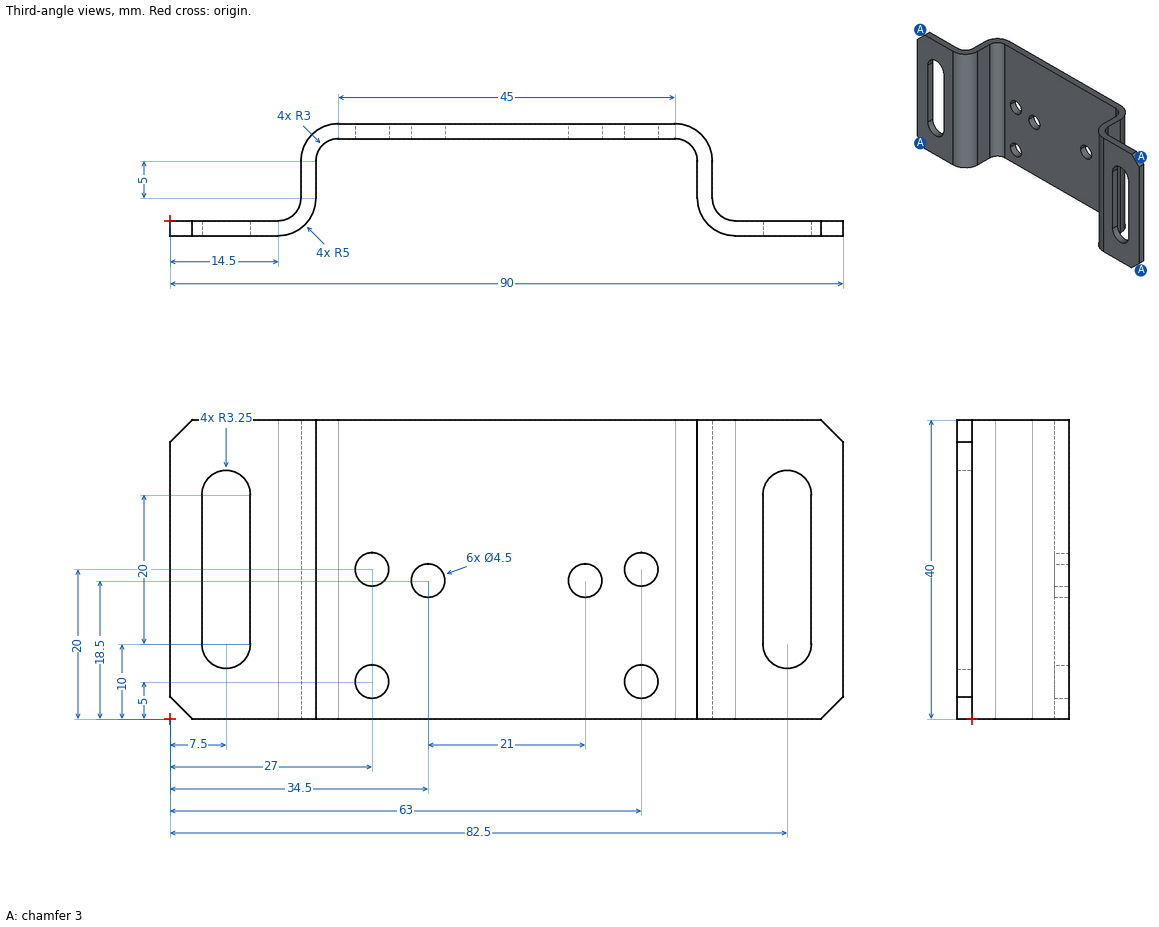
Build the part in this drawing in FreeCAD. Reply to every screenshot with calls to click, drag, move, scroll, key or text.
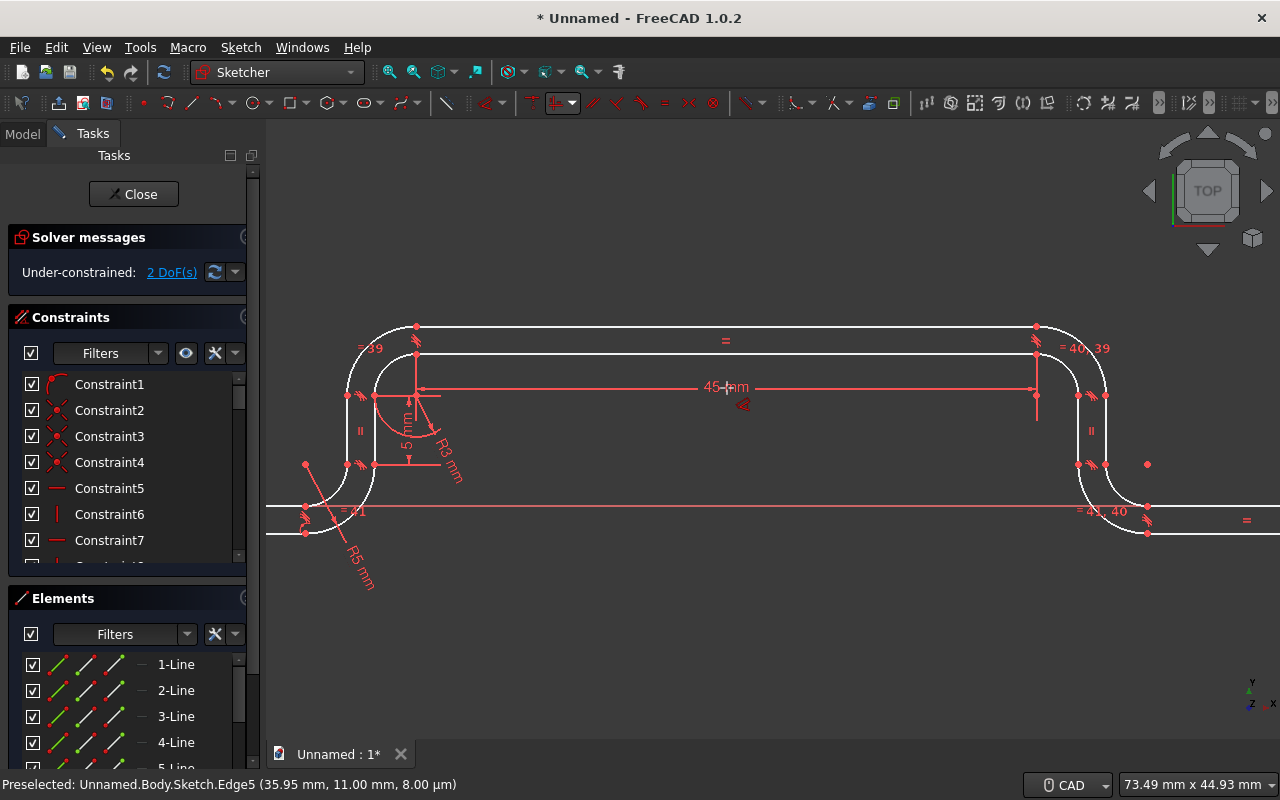
scroll(686, 428, down, 4)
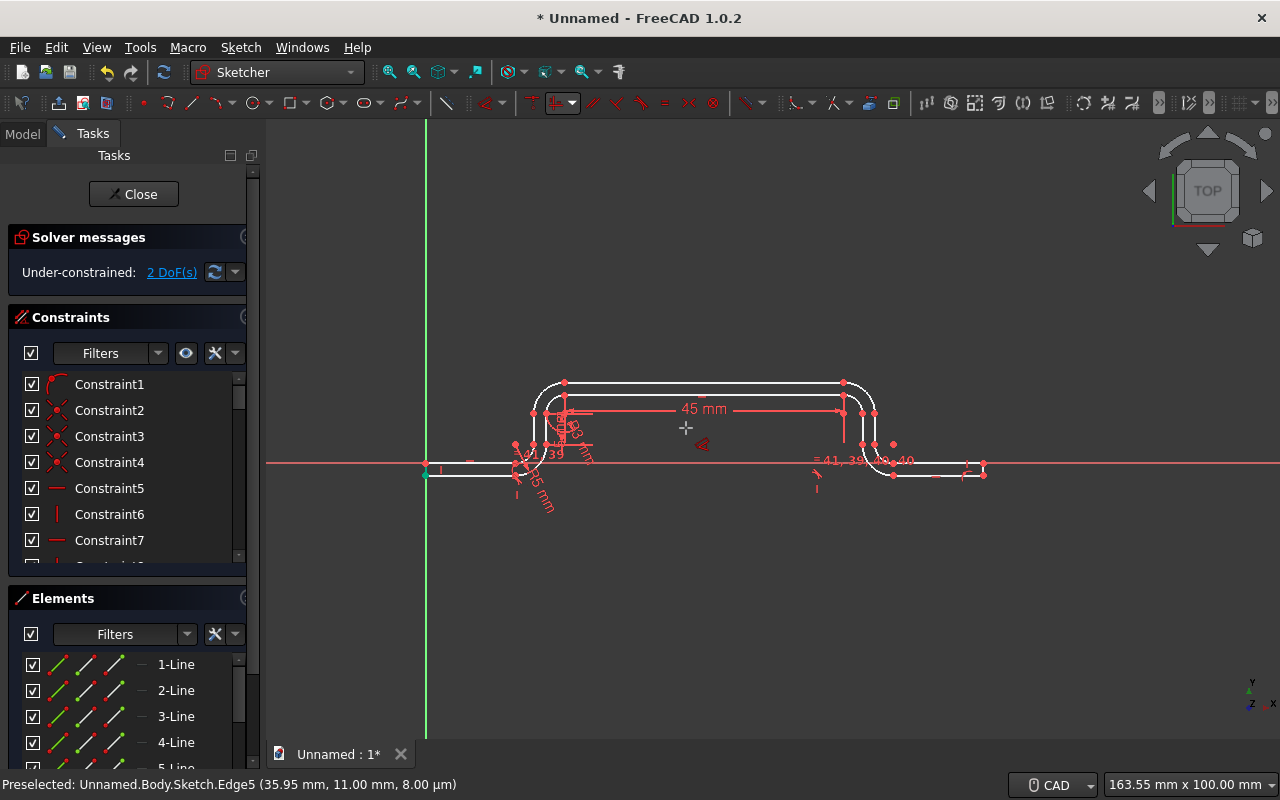
click(983, 476)
click(704, 510)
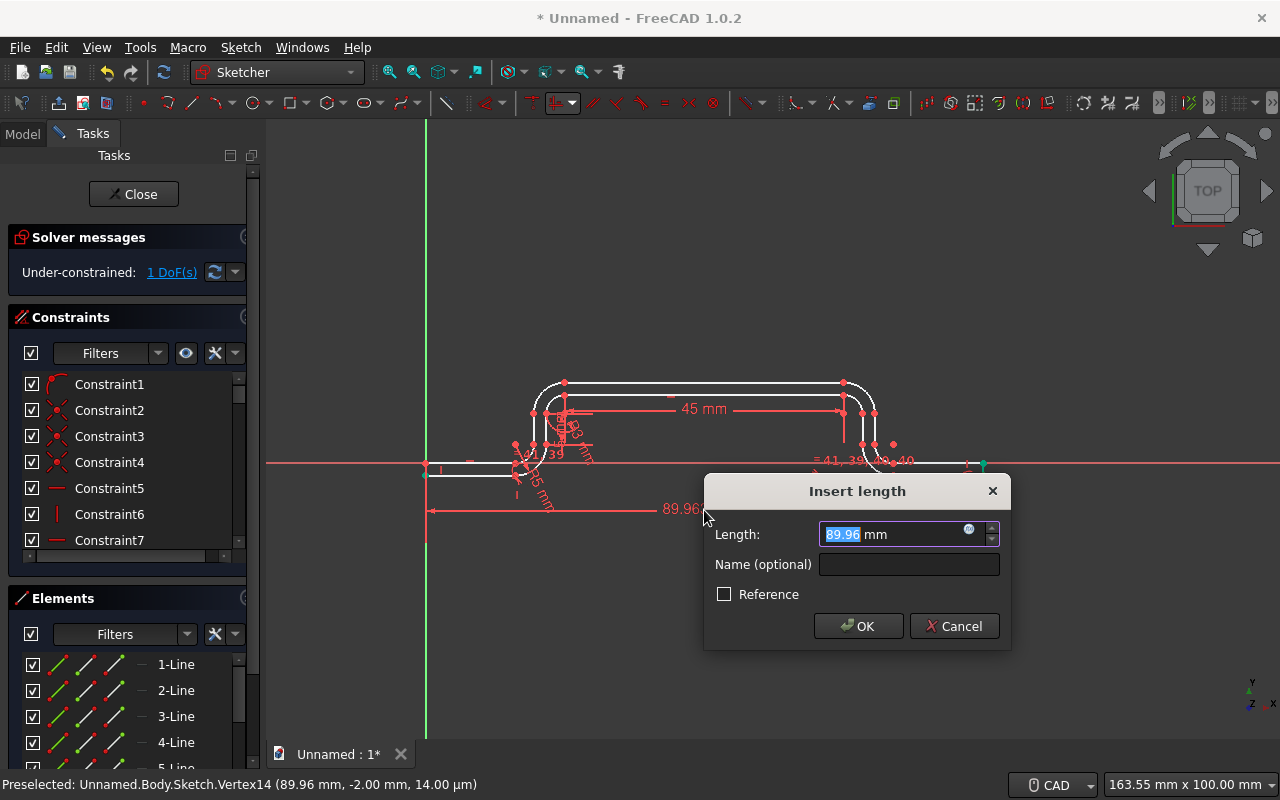
text(90)
key(Return)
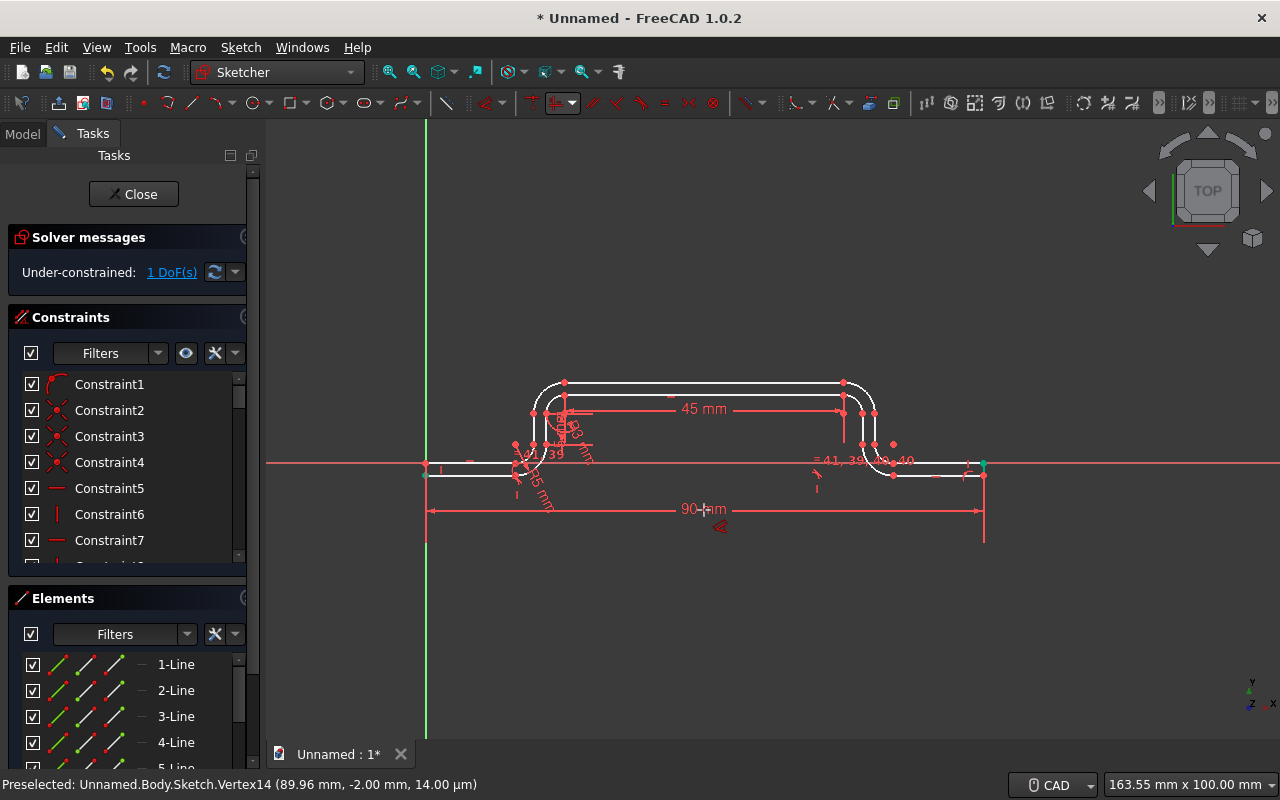
click(488, 463)
click(450, 497)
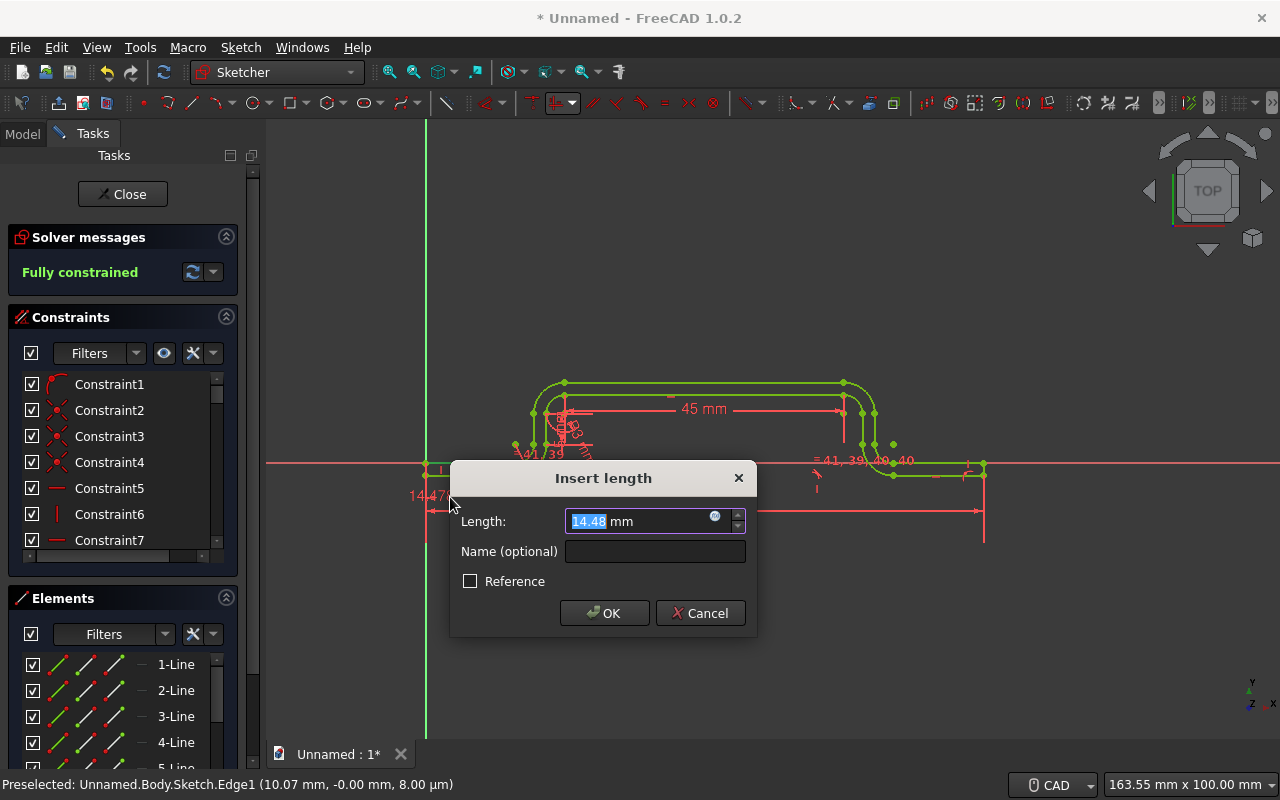
text(14.5)
key(Return)
key(Escape)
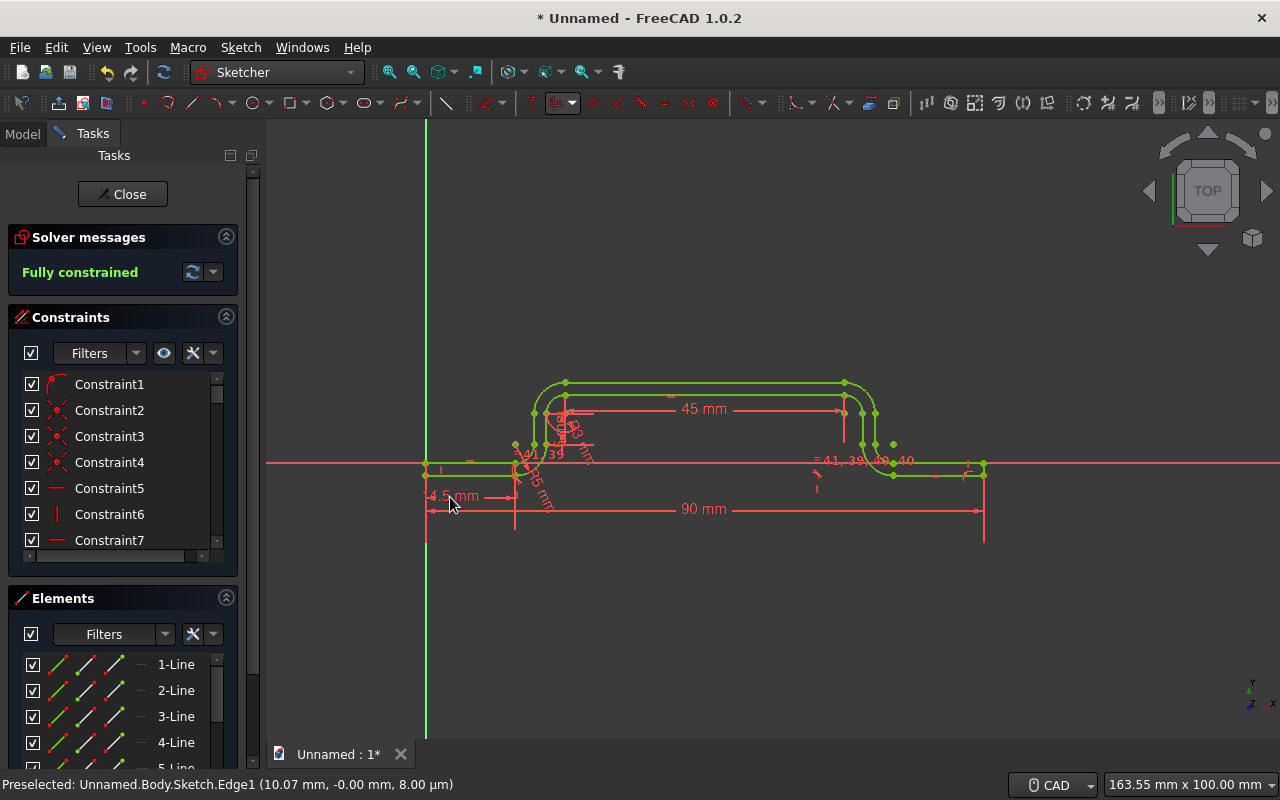
click(123, 194)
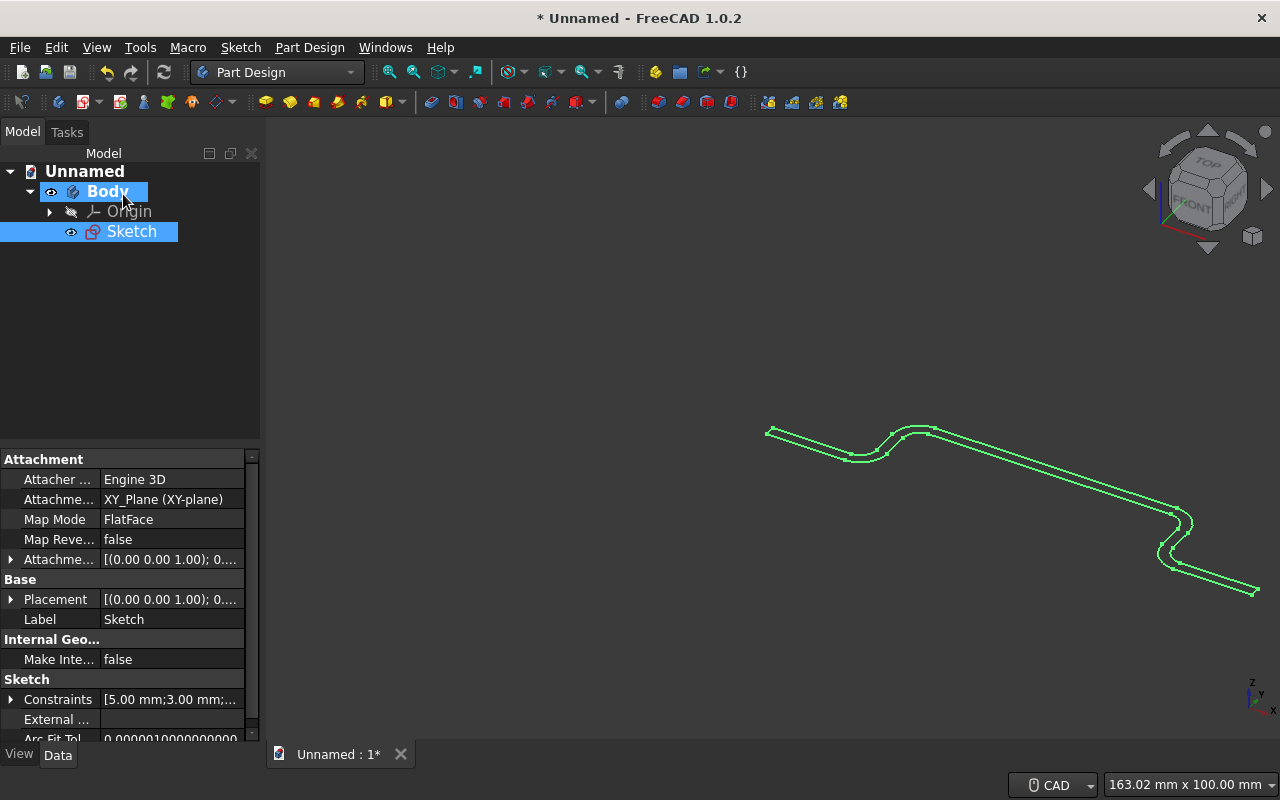
click(266, 102)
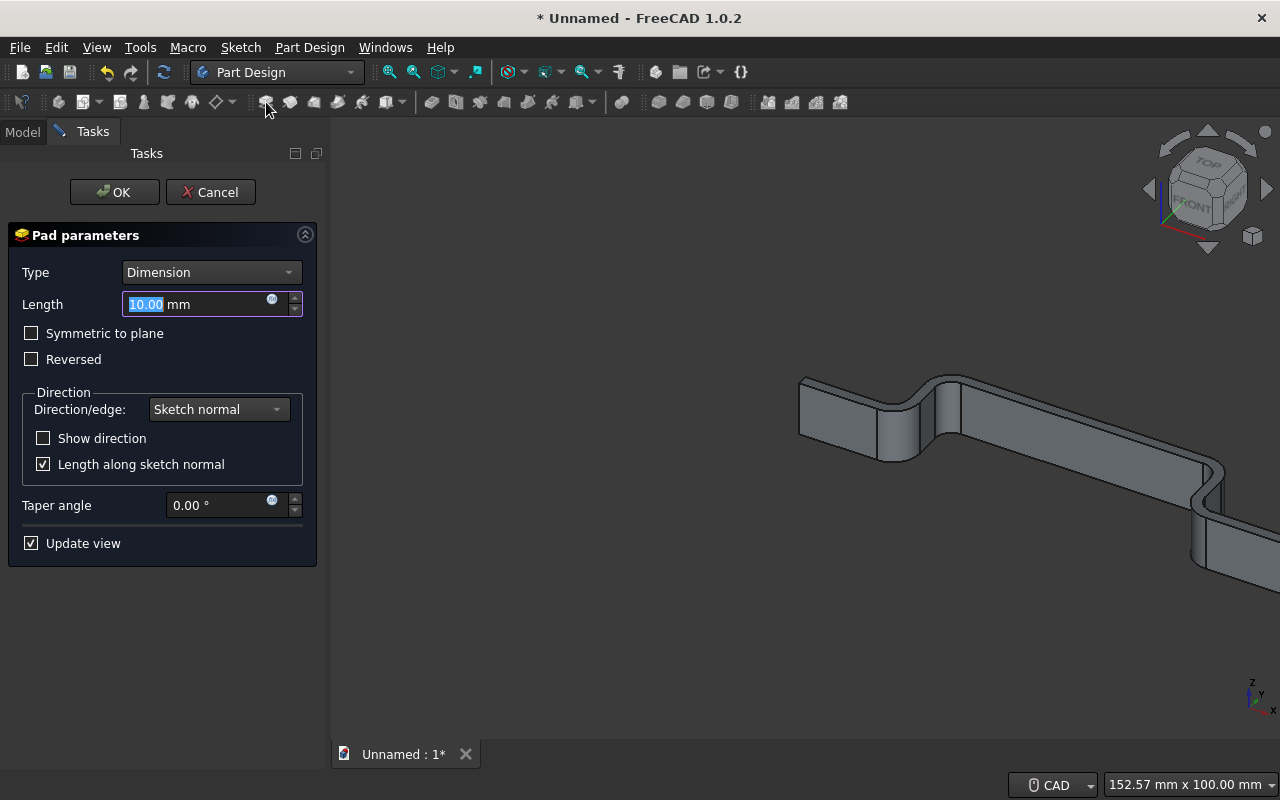
text(40)
key(Tab)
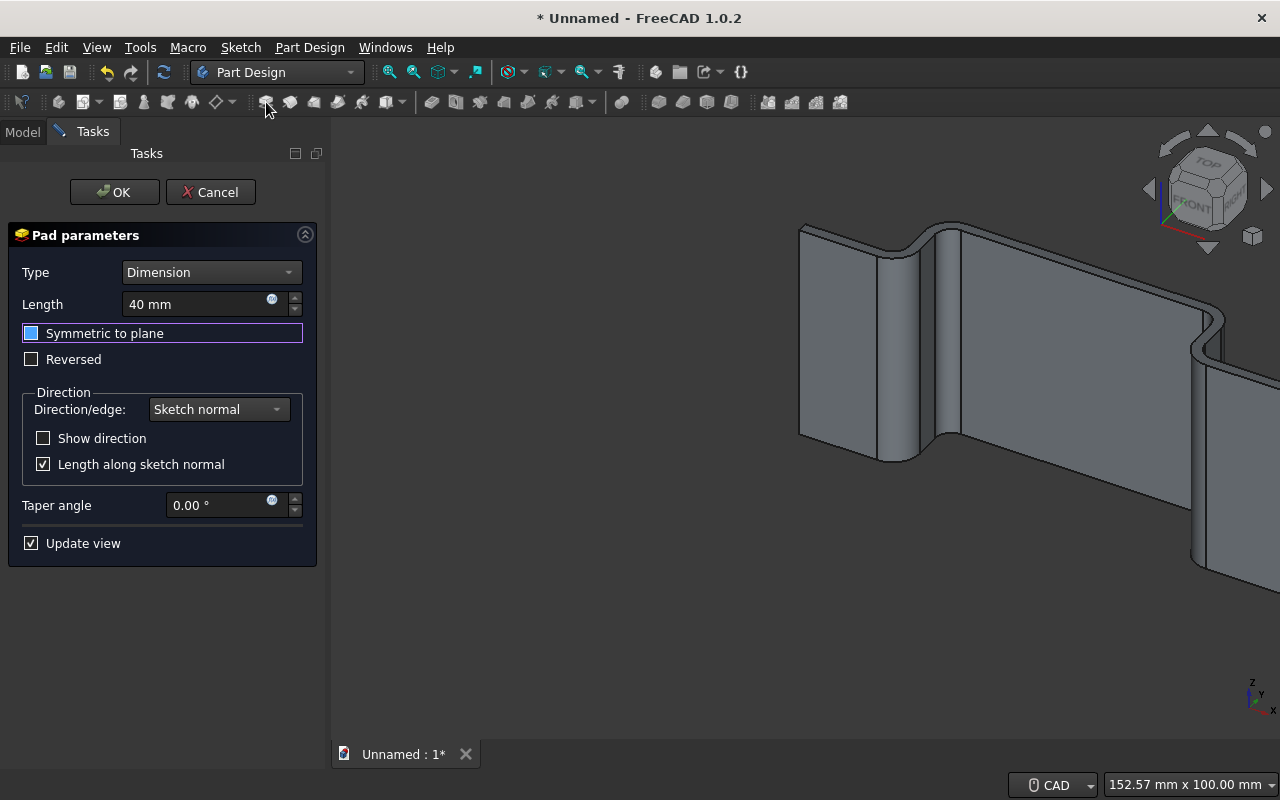
click(115, 192)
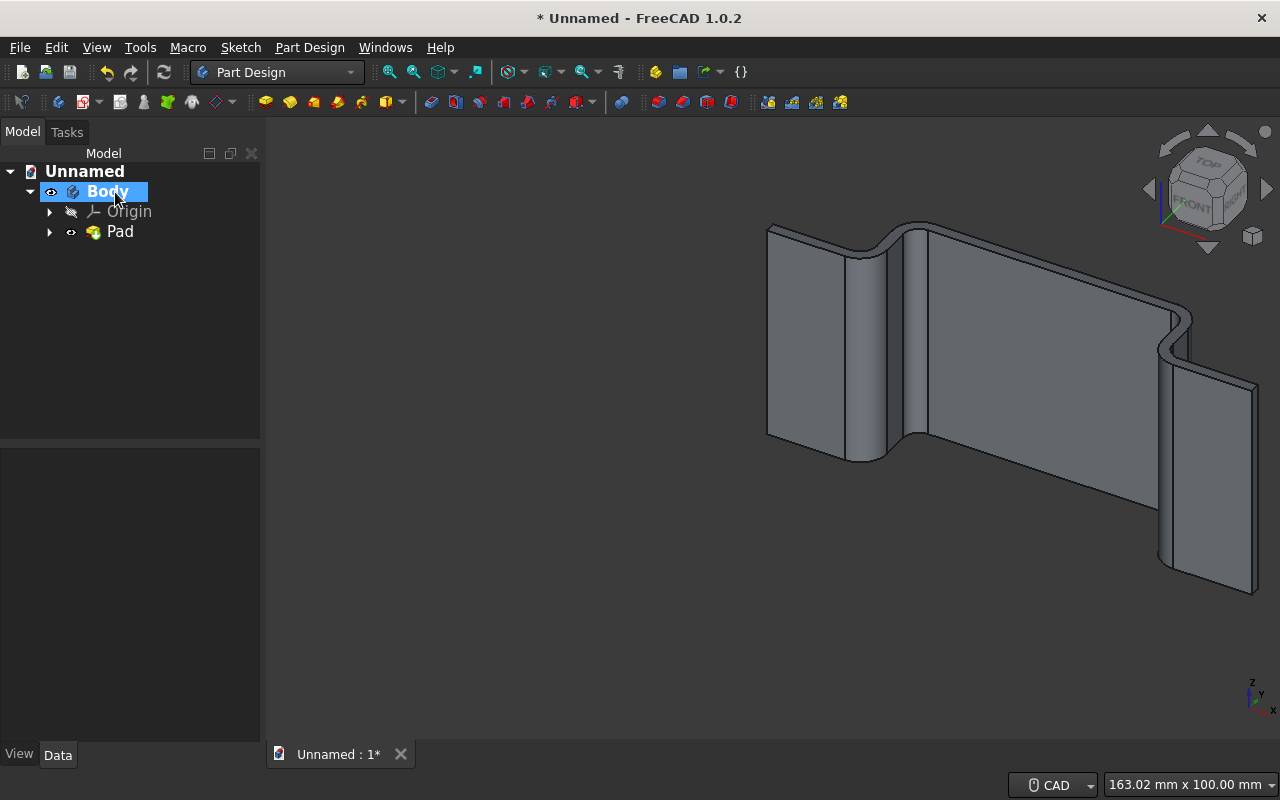
key(v)
key(f)